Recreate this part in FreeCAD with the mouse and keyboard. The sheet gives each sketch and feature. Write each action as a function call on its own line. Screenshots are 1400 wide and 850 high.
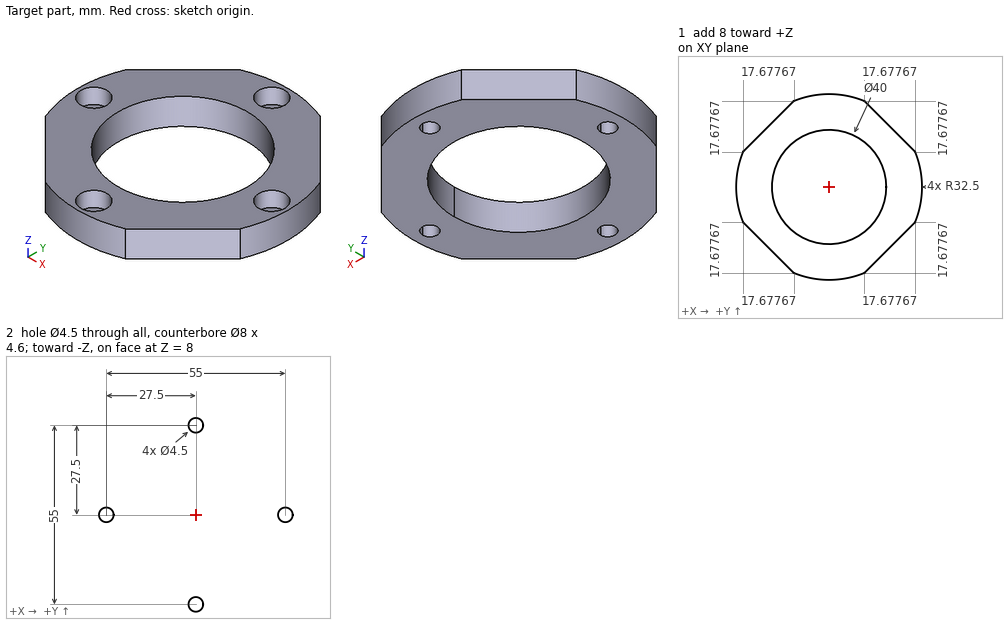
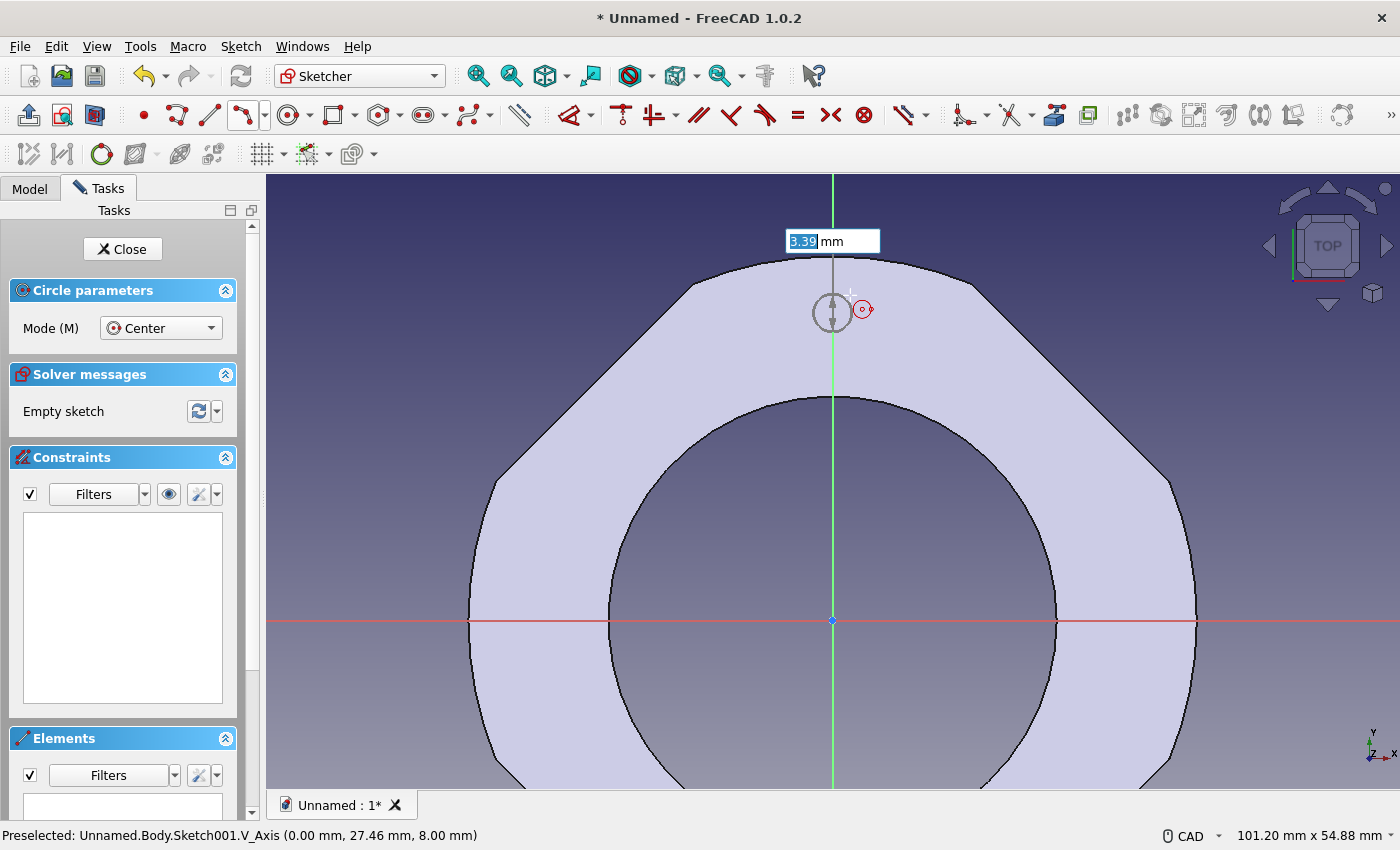
text(4.5)
key(Return)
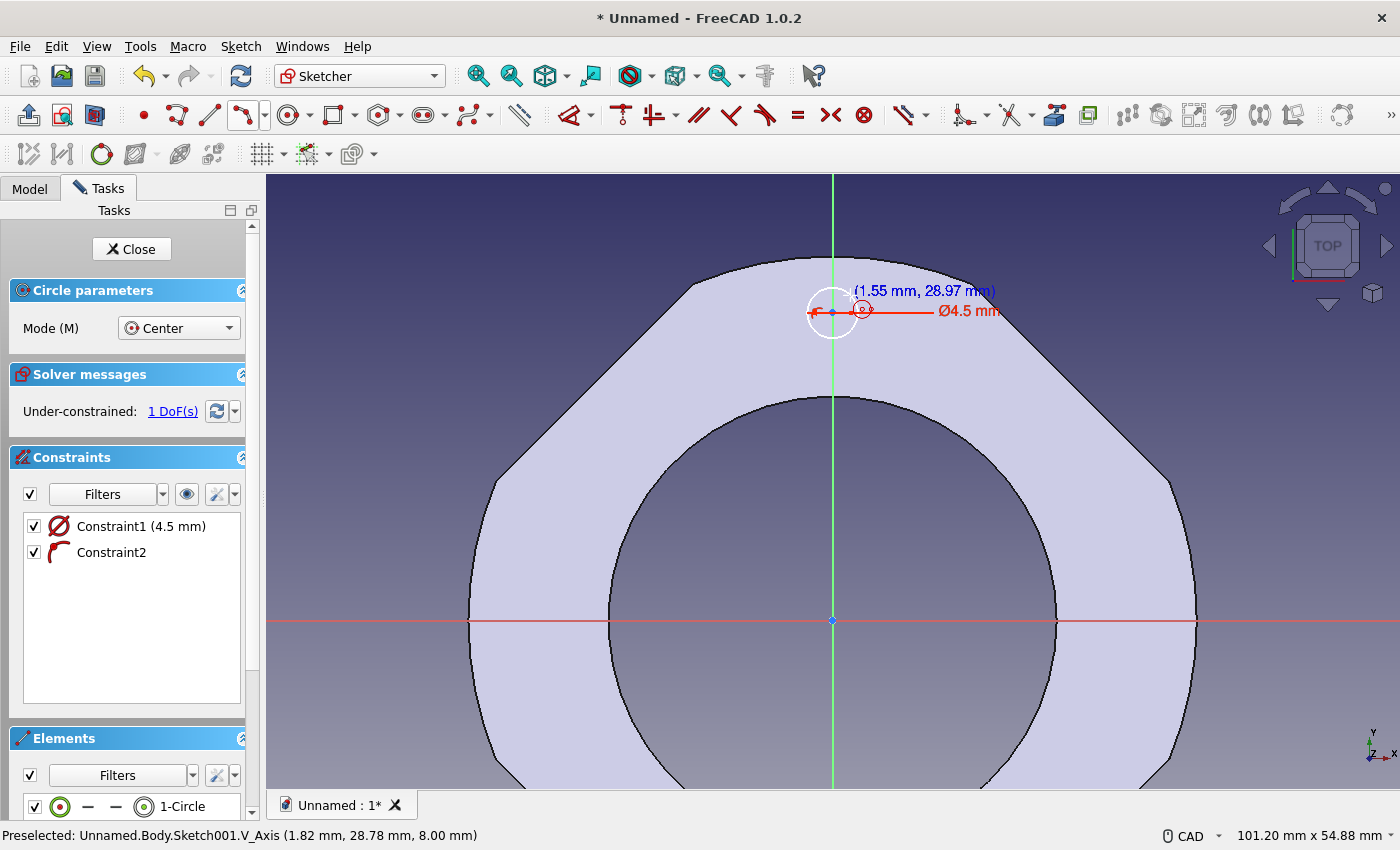
click(524, 621)
move(542, 603)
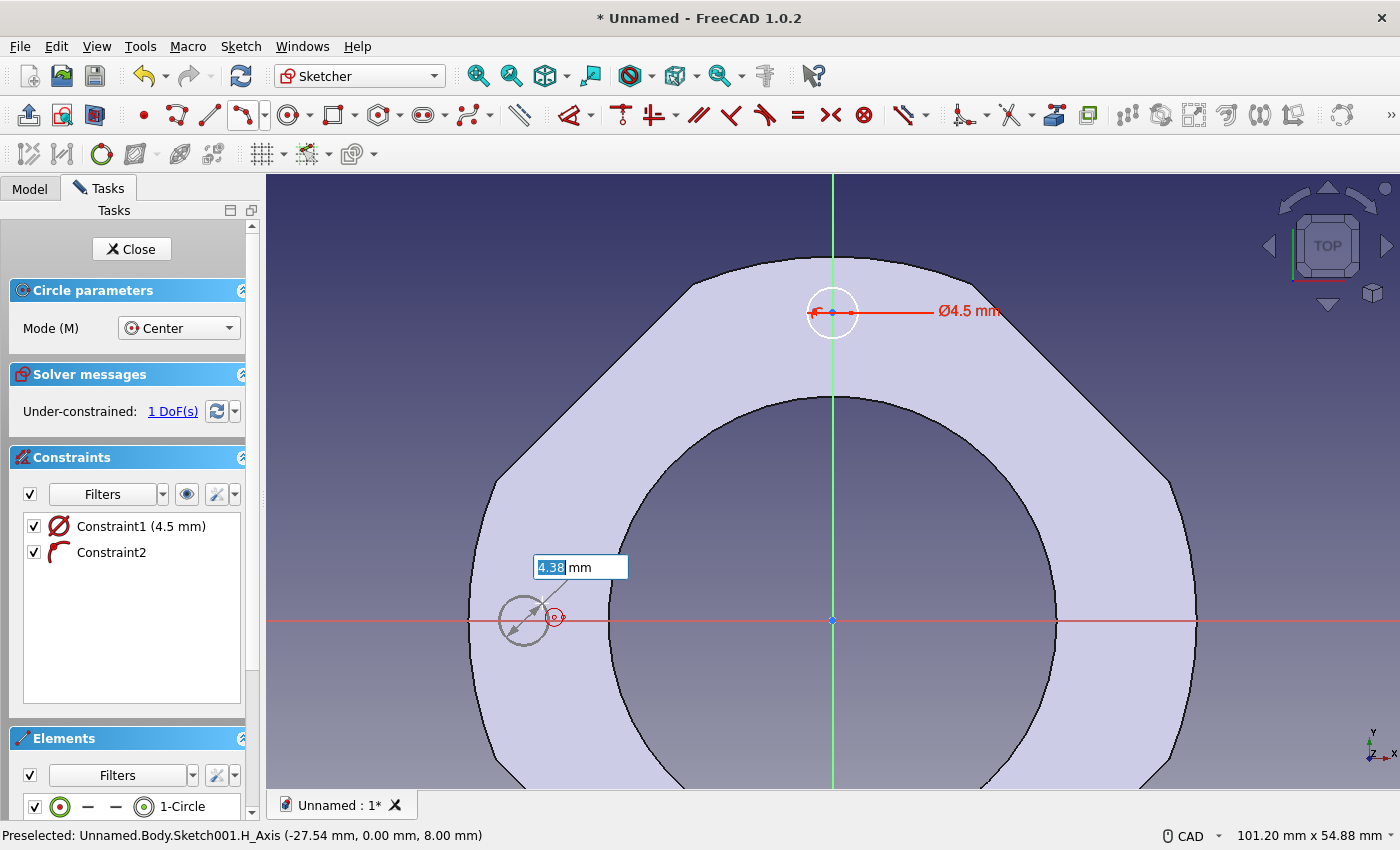
text(4.5)
key(Return)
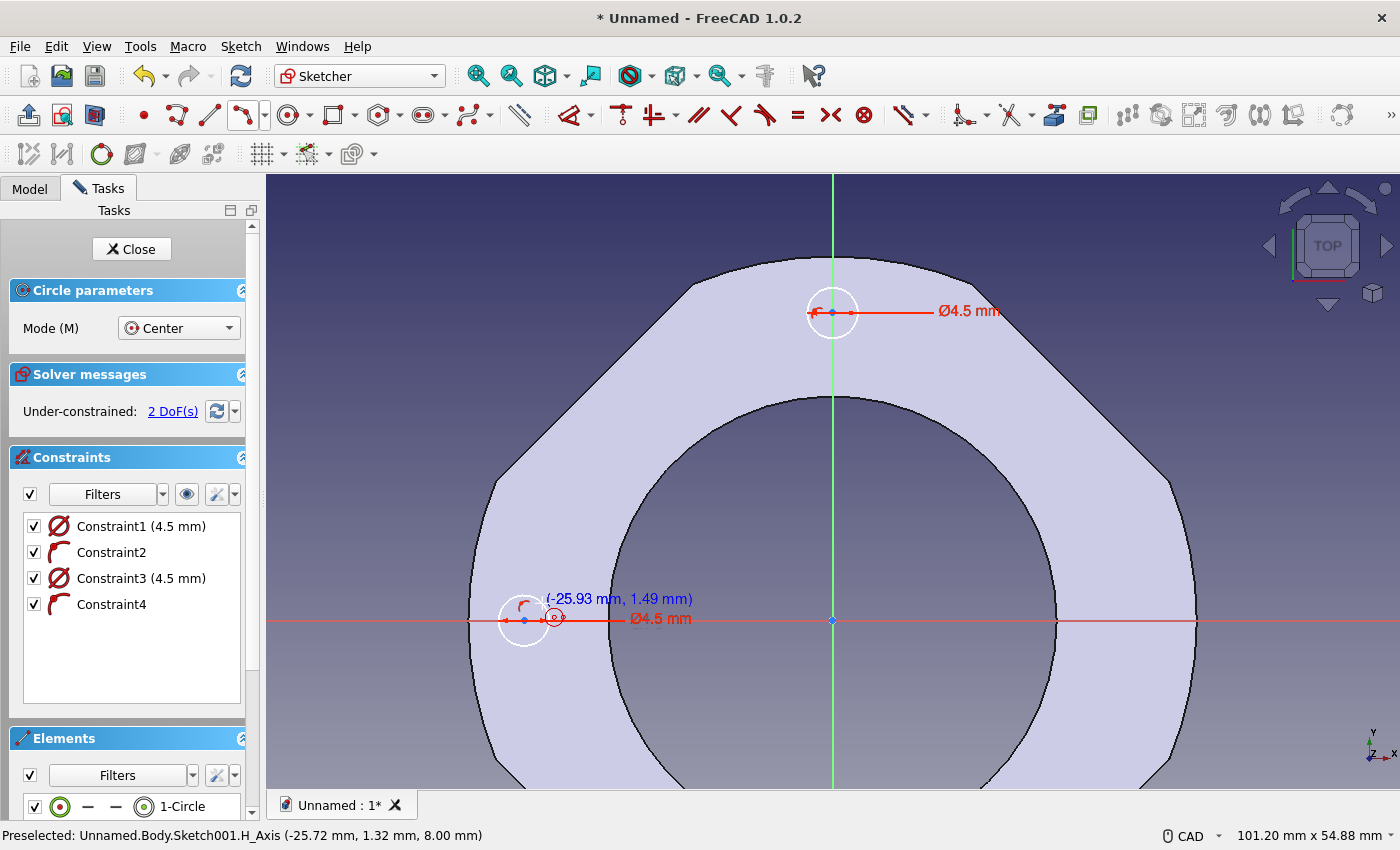
scroll(682, 312, down, 3)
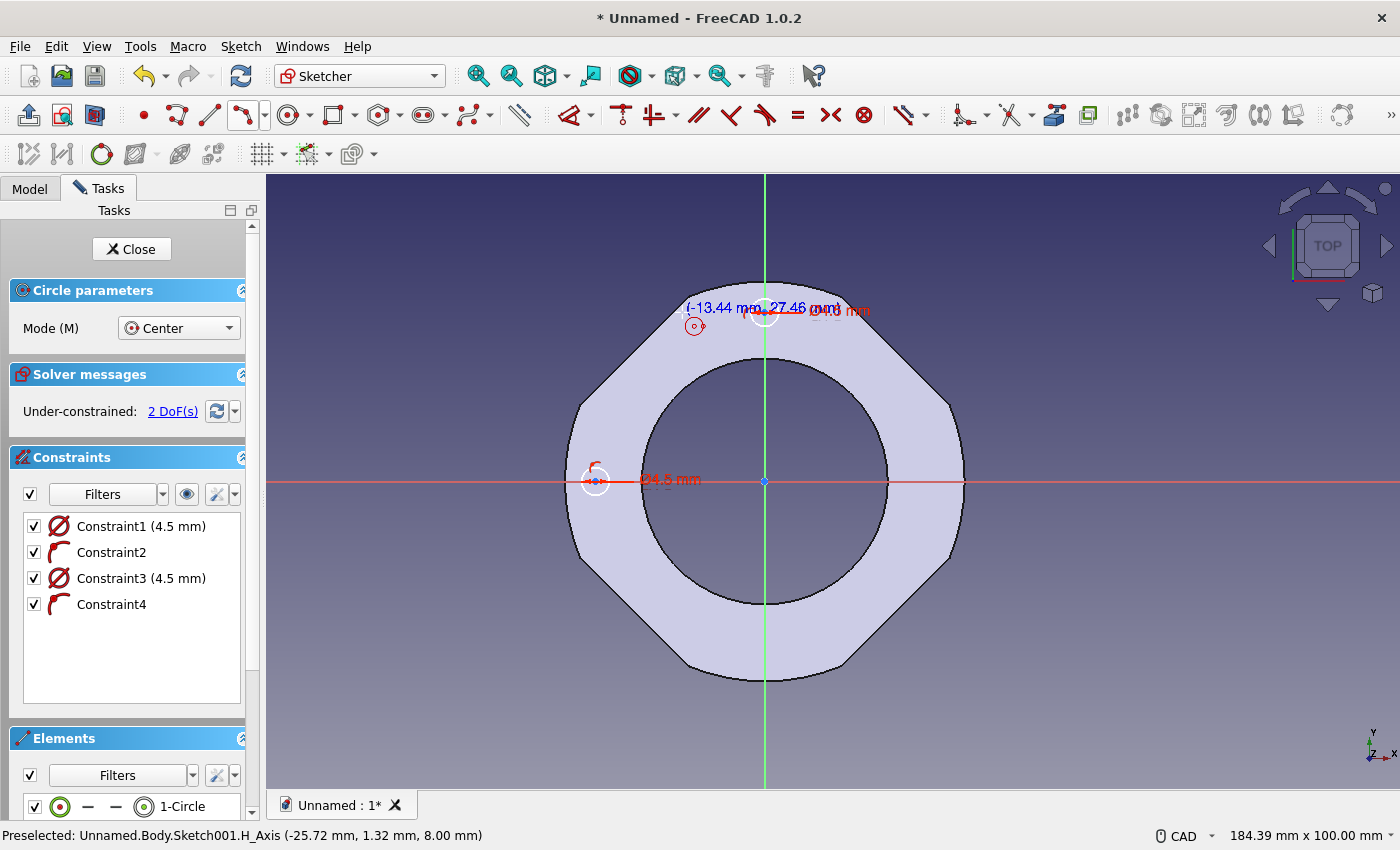
scroll(765, 651, up, 3)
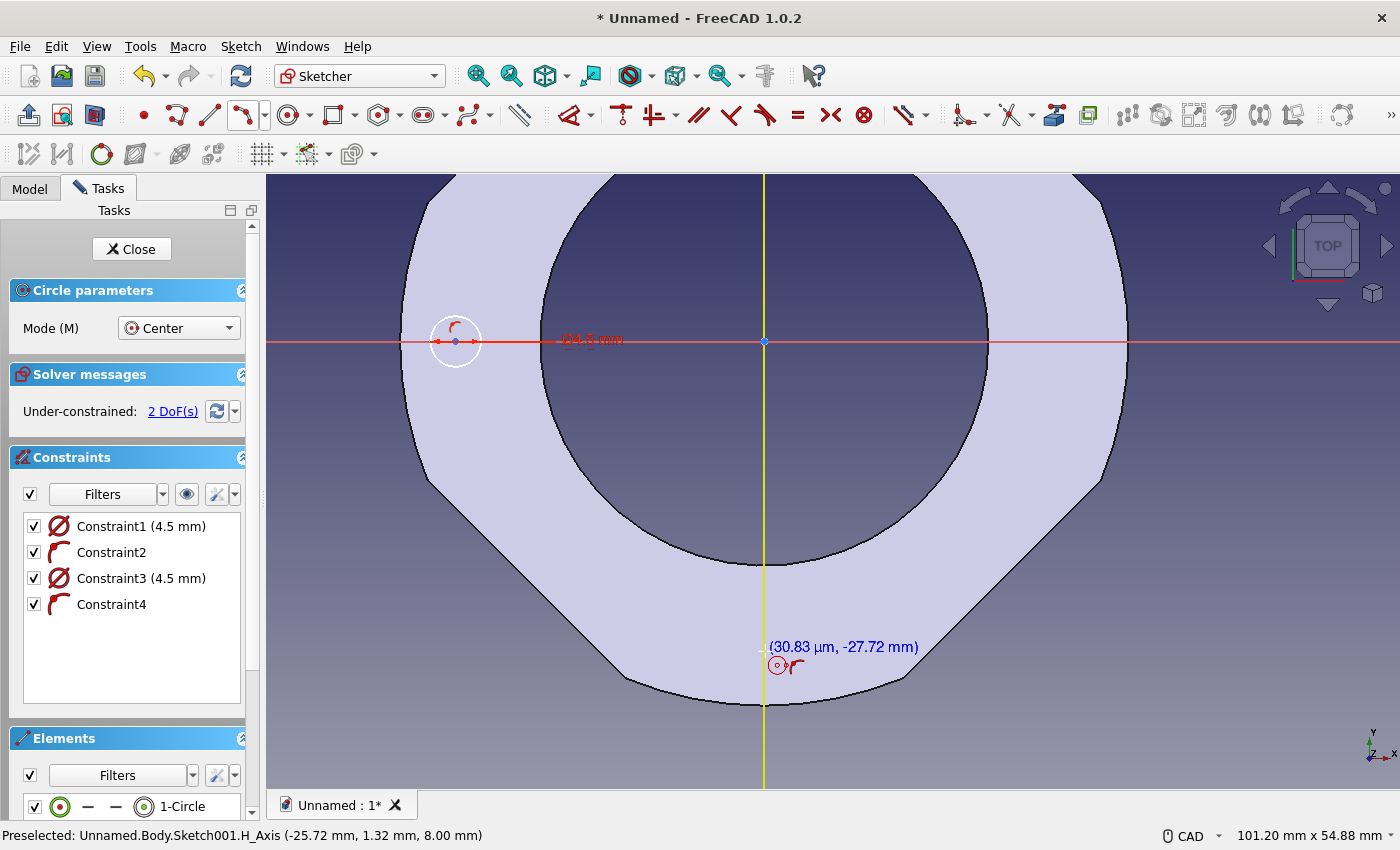
click(764, 650)
move(782, 632)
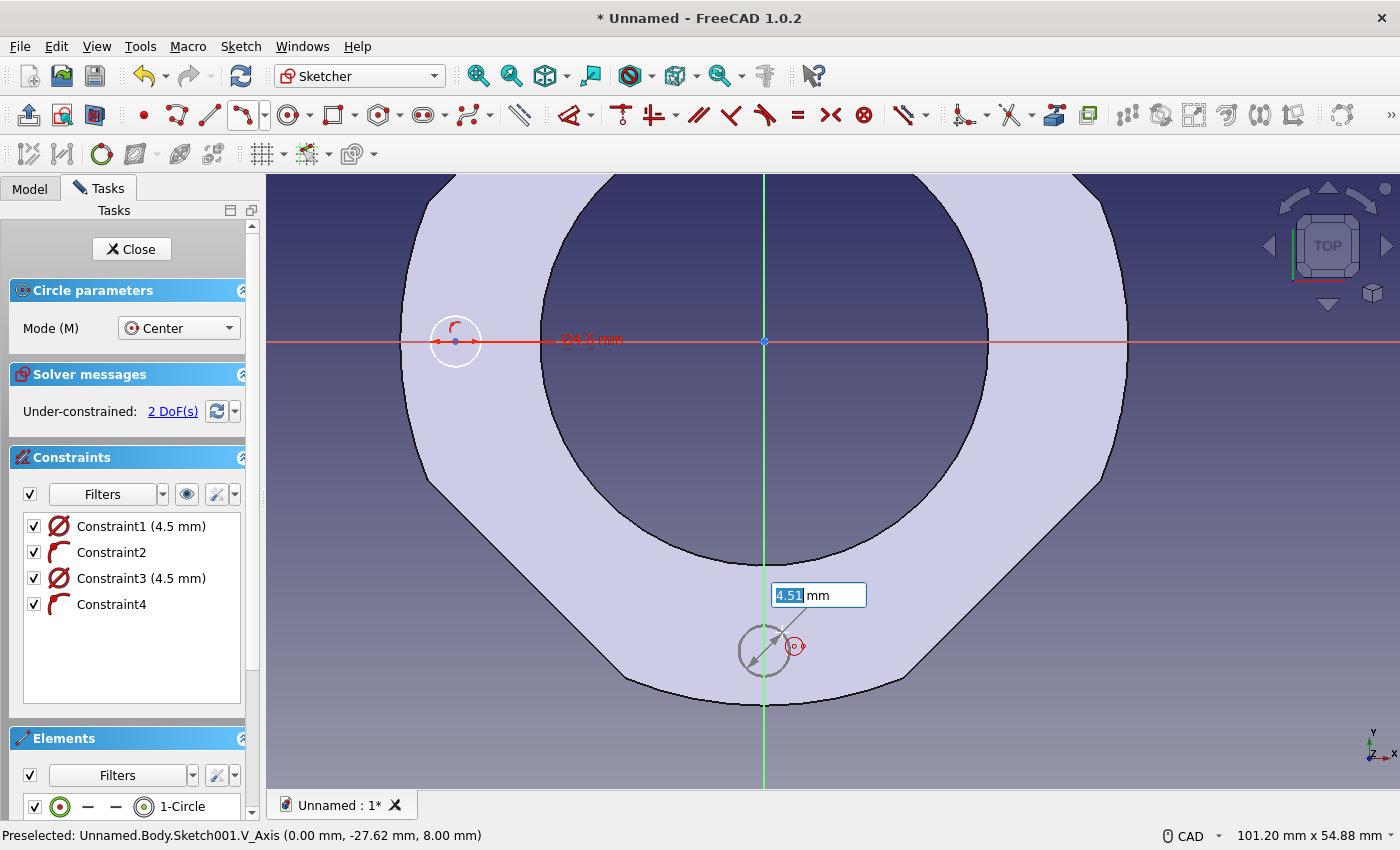
text(4.5)
key(Return)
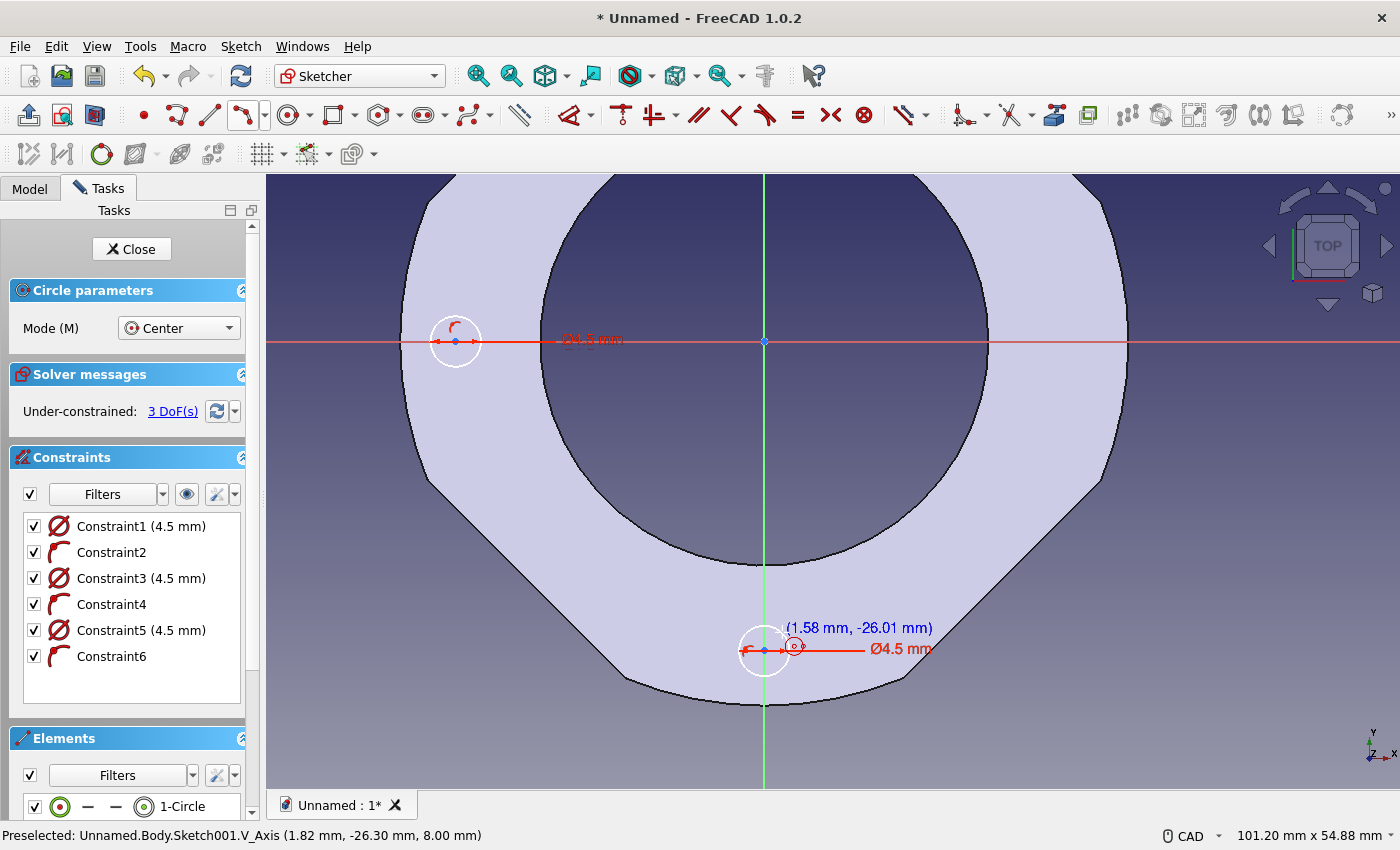
click(1072, 342)
move(1090, 324)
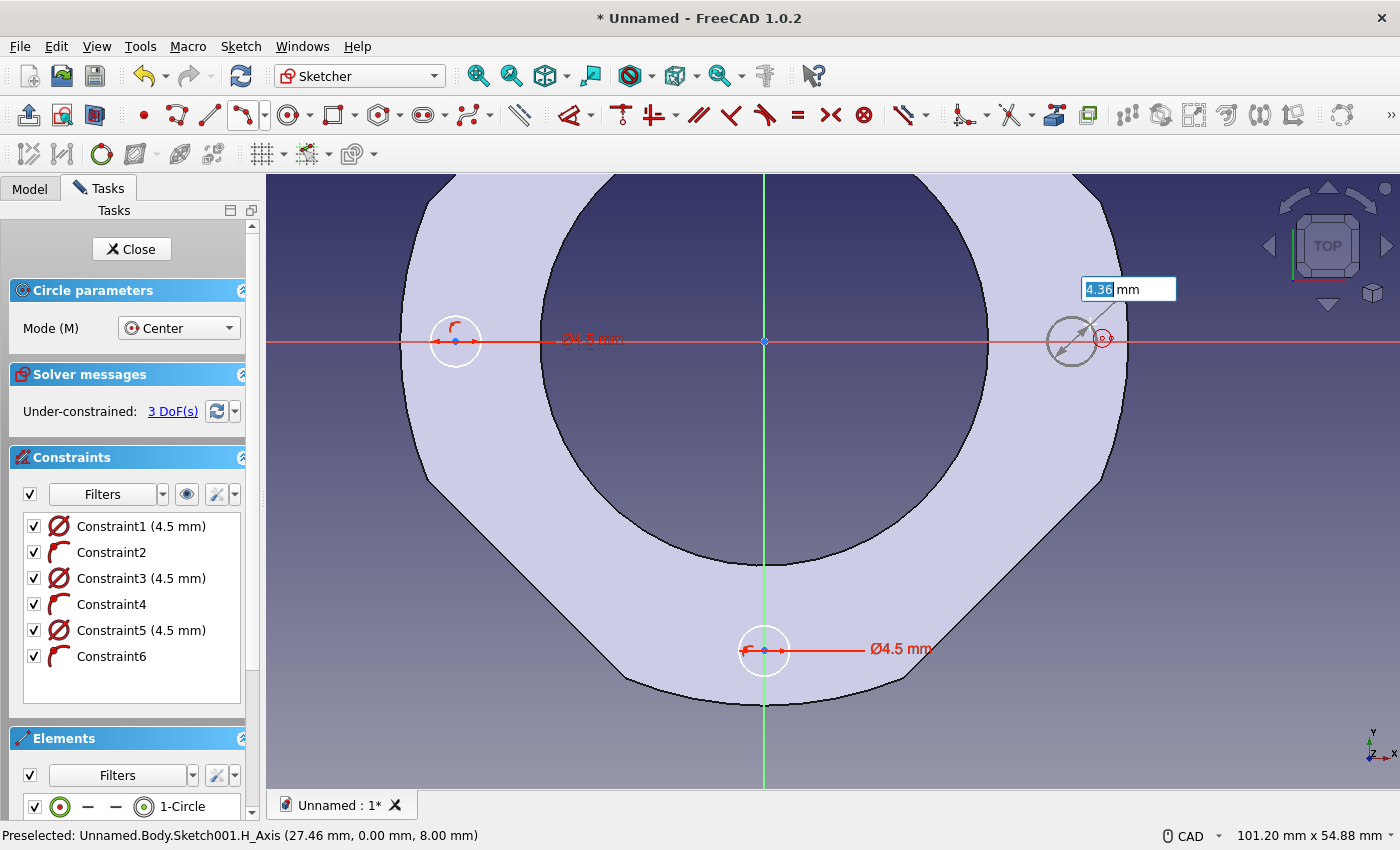
text(4.5)
key(Return)
key(Escape)